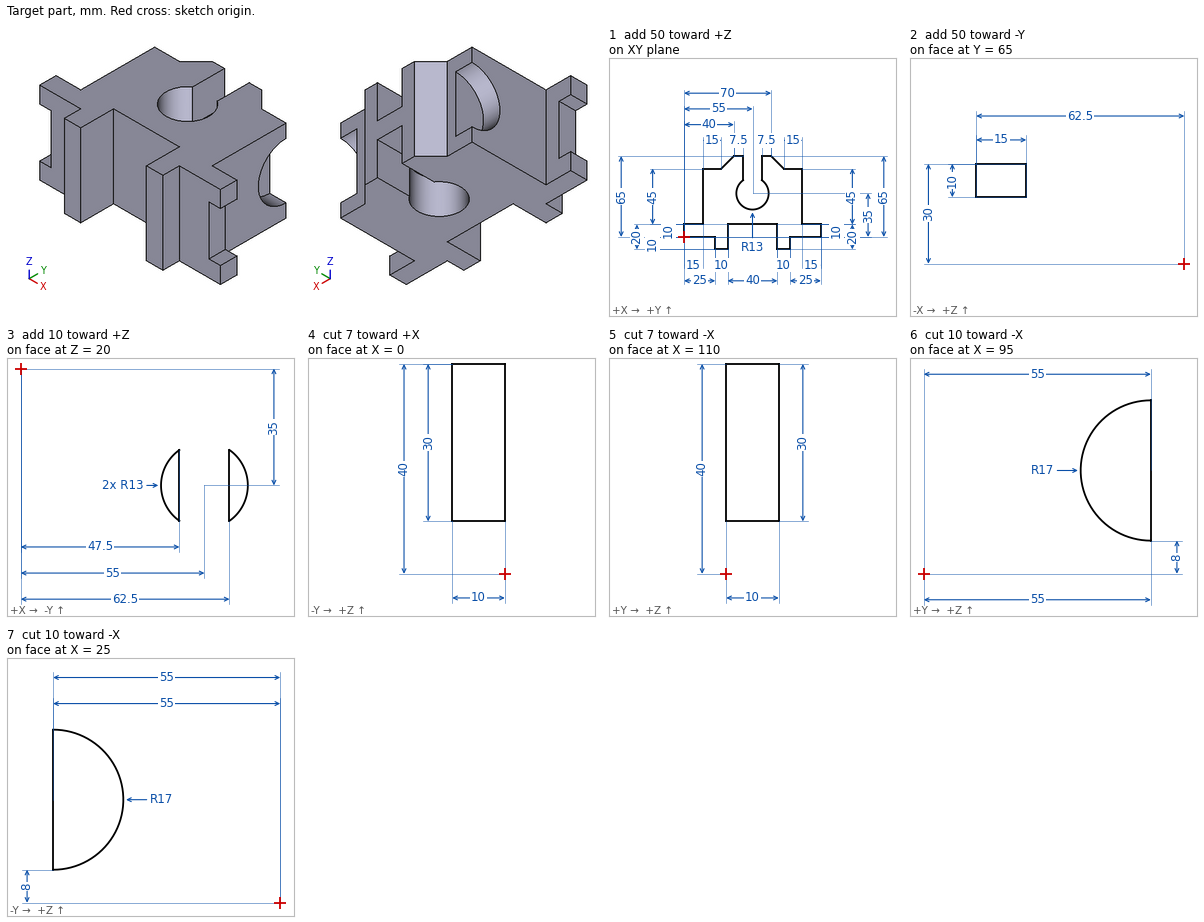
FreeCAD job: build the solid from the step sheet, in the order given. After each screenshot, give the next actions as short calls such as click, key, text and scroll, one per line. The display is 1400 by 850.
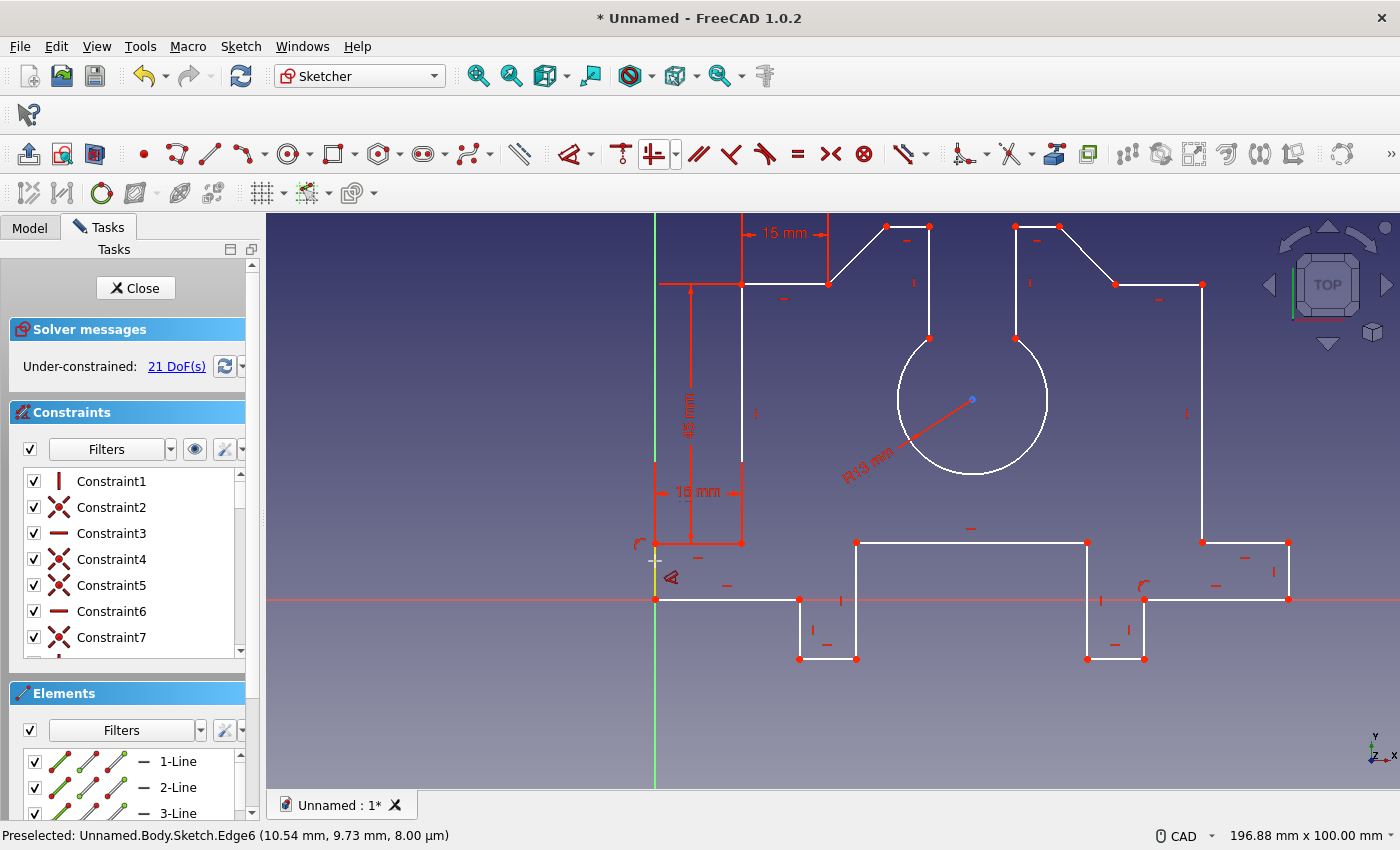
click(655, 560)
click(621, 572)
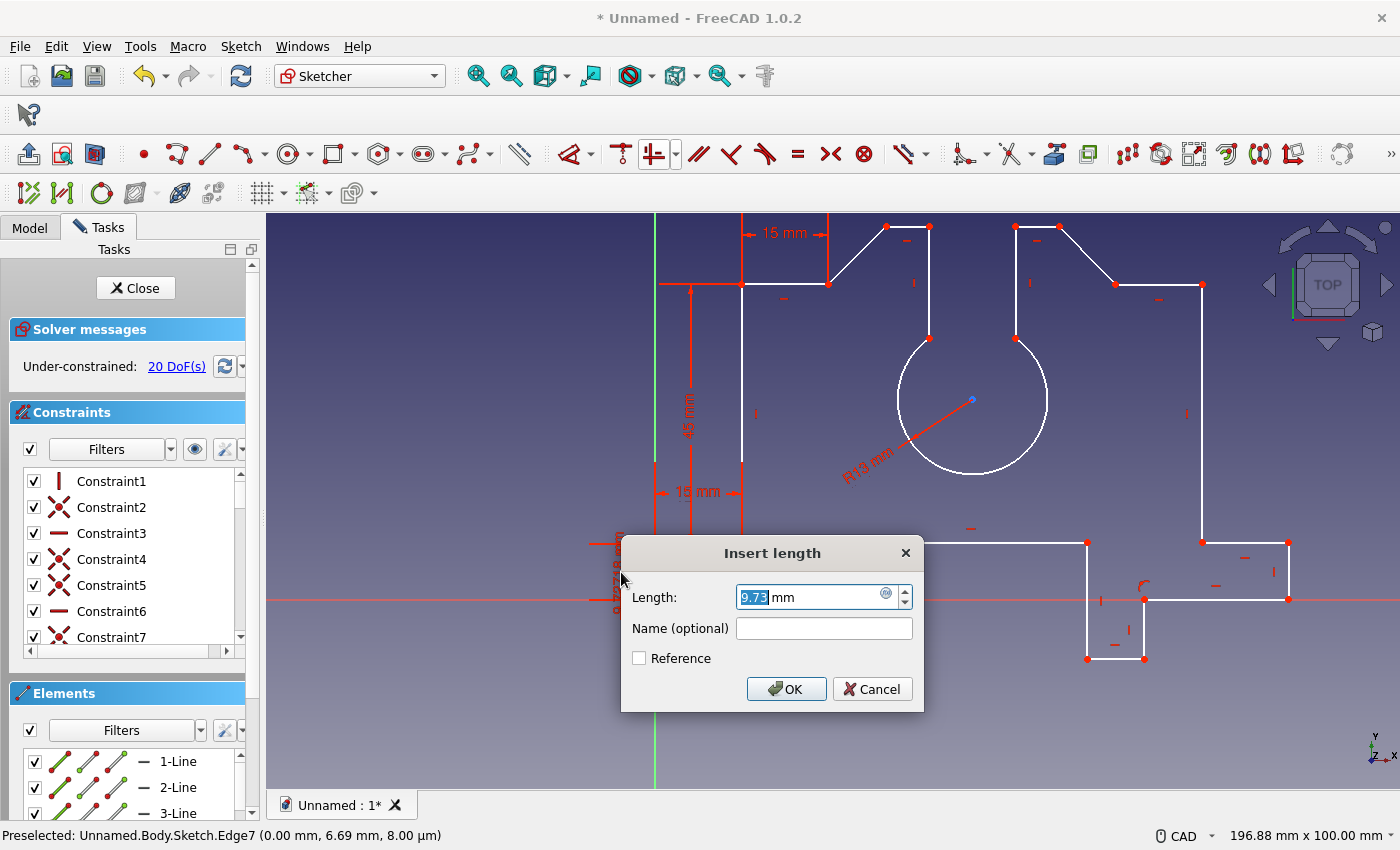
text(10)
key(Return)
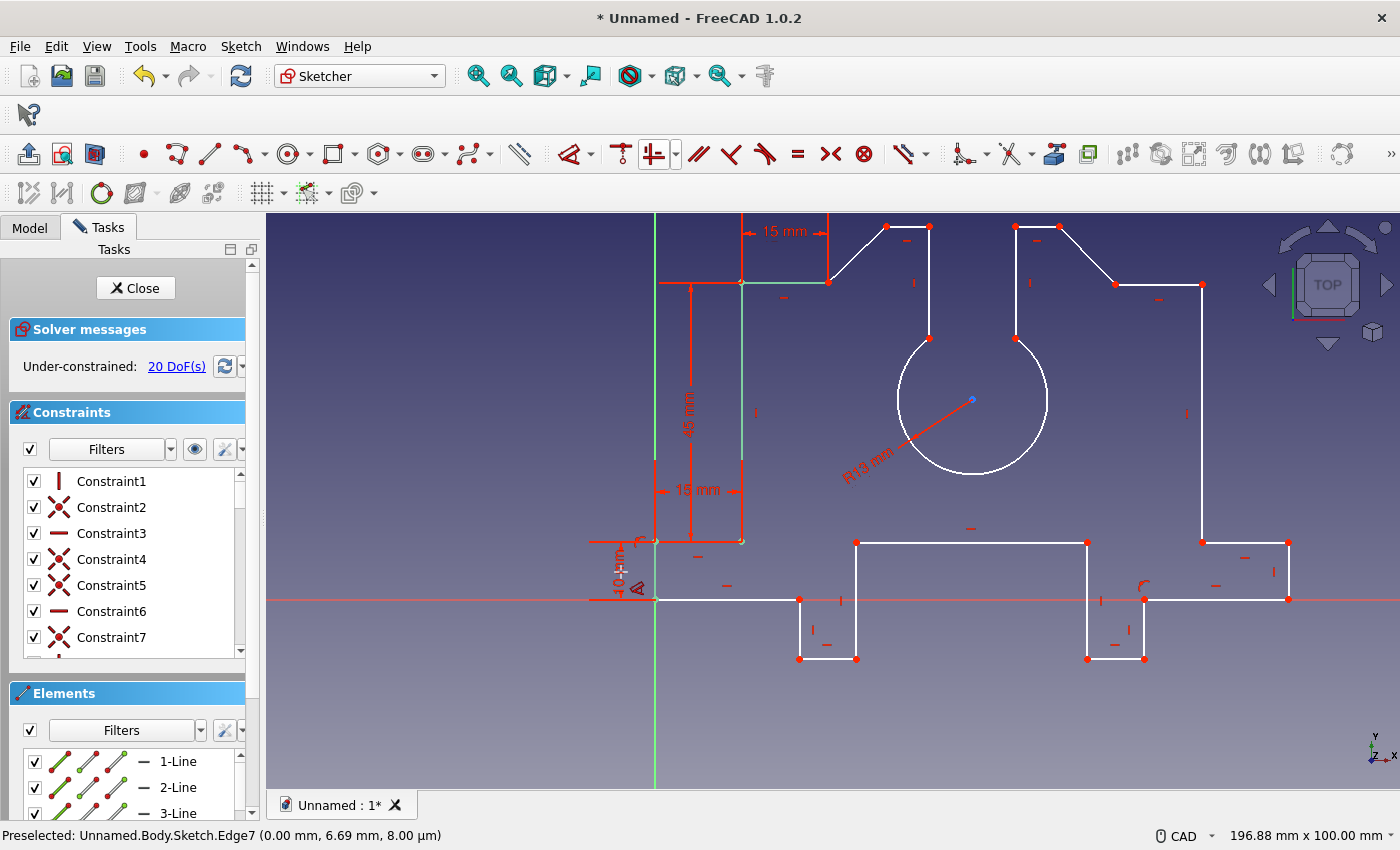
click(699, 600)
click(727, 634)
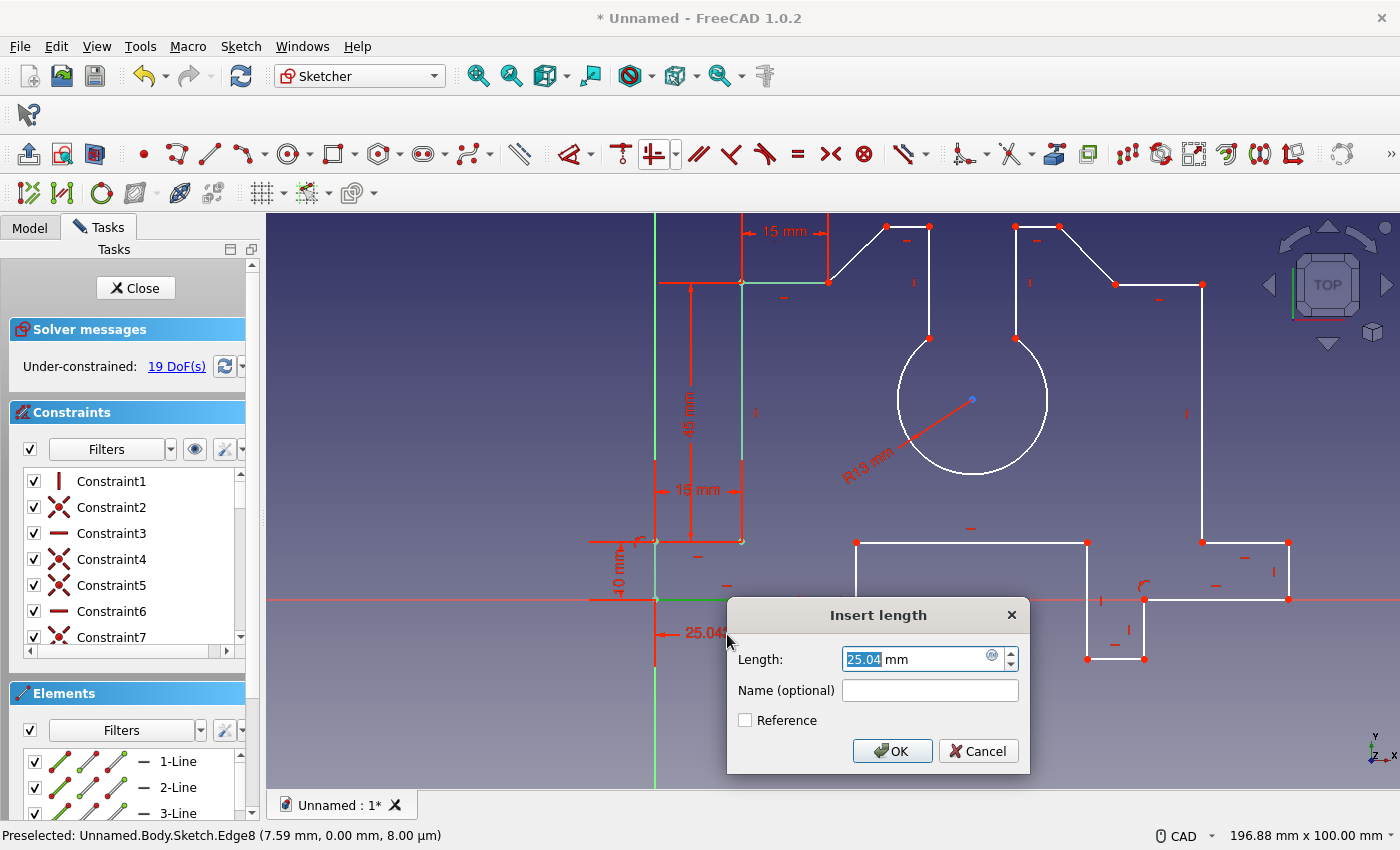
text(25)
key(Return)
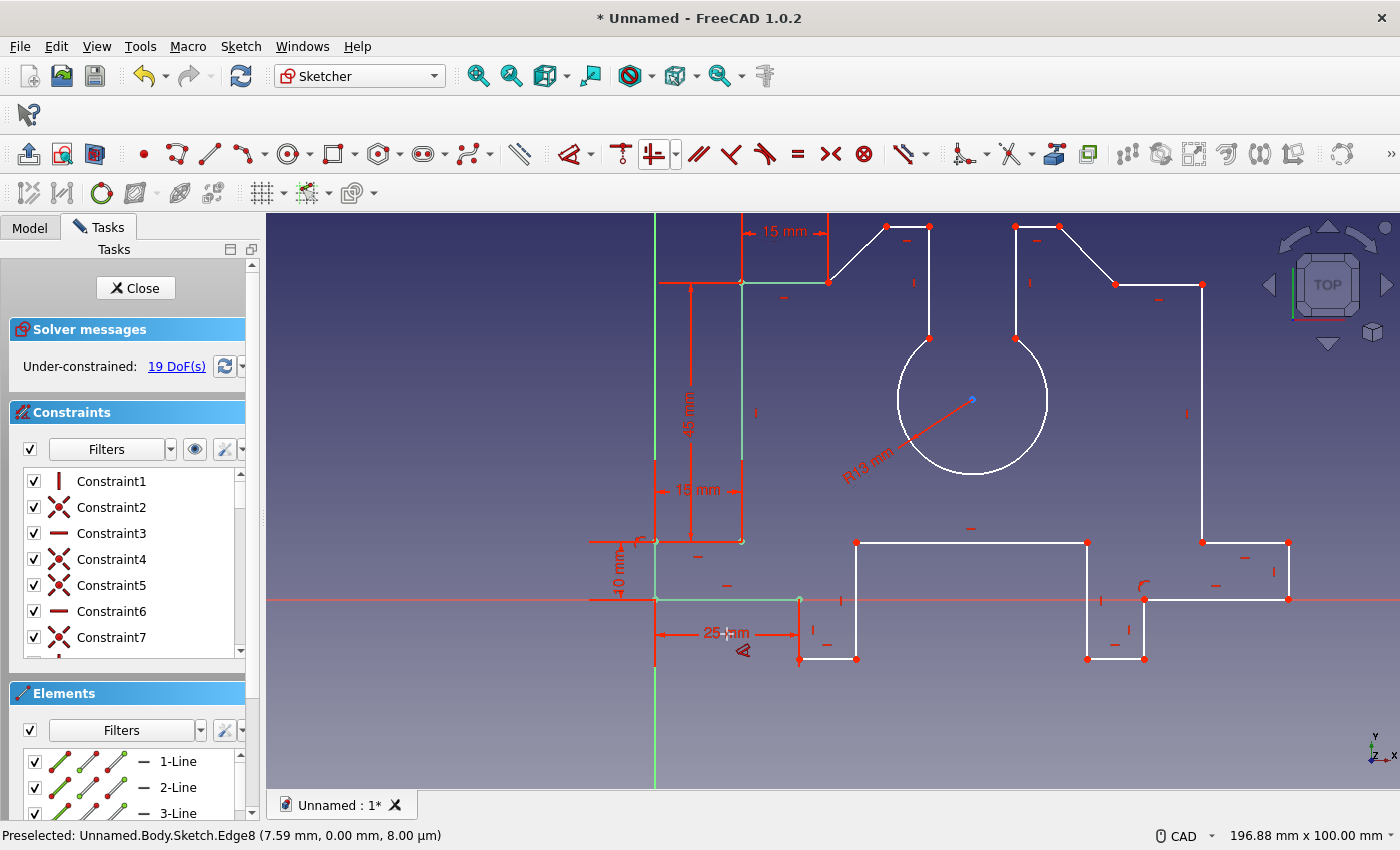
click(799, 617)
click(833, 629)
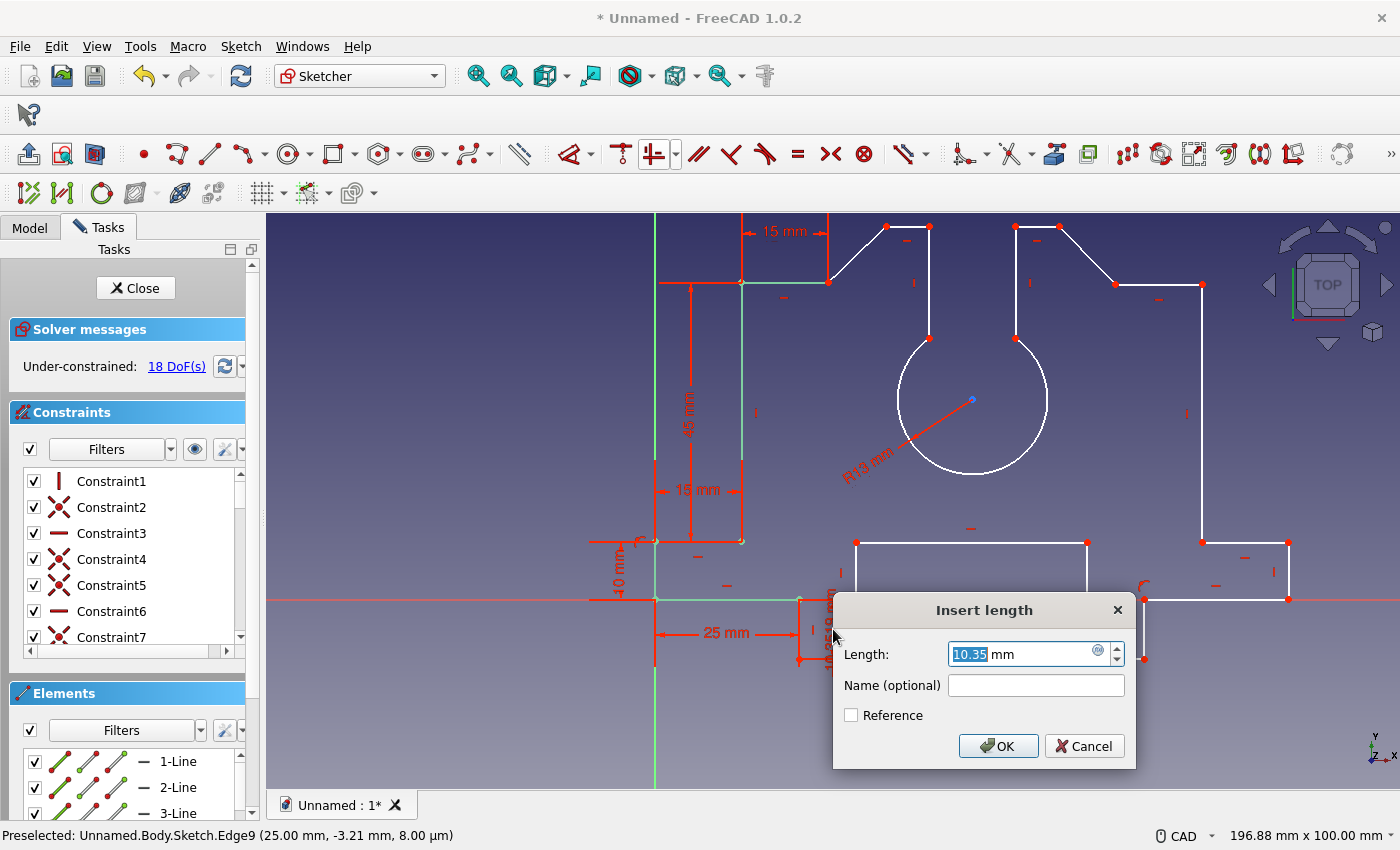
text(10)
key(Return)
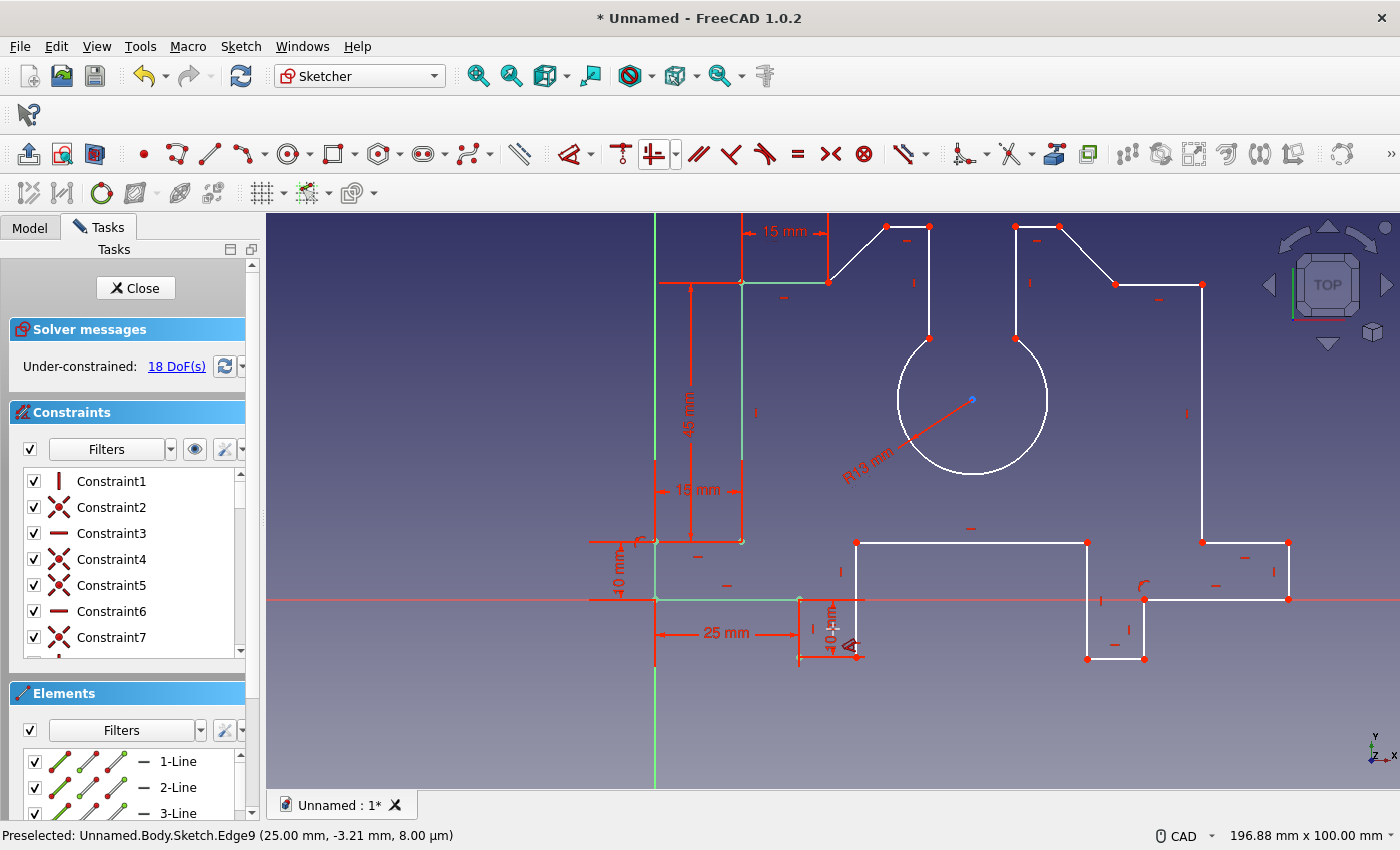
click(816, 657)
click(828, 691)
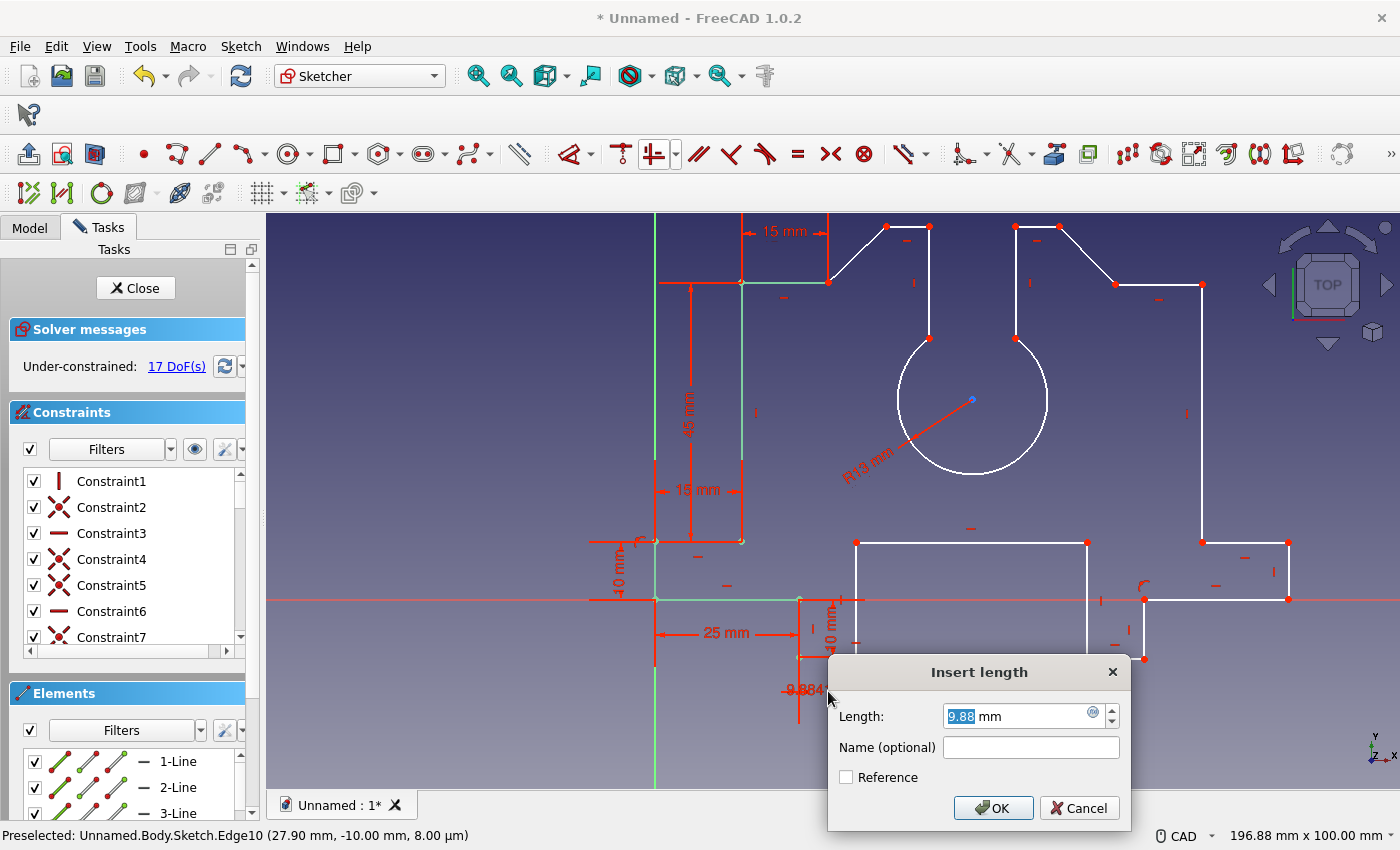
text(10)
key(Return)